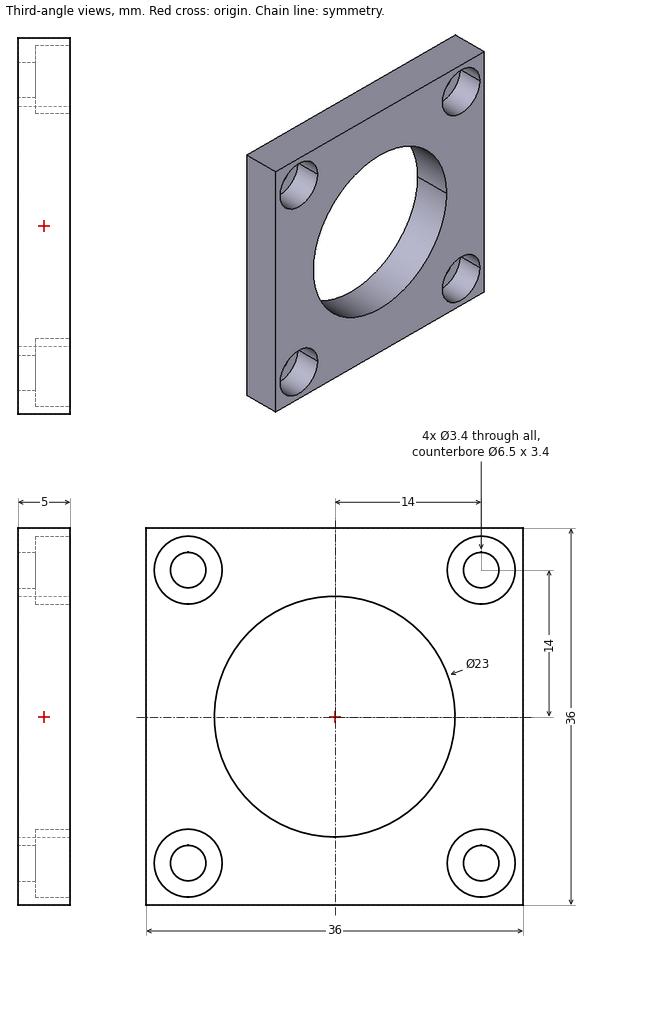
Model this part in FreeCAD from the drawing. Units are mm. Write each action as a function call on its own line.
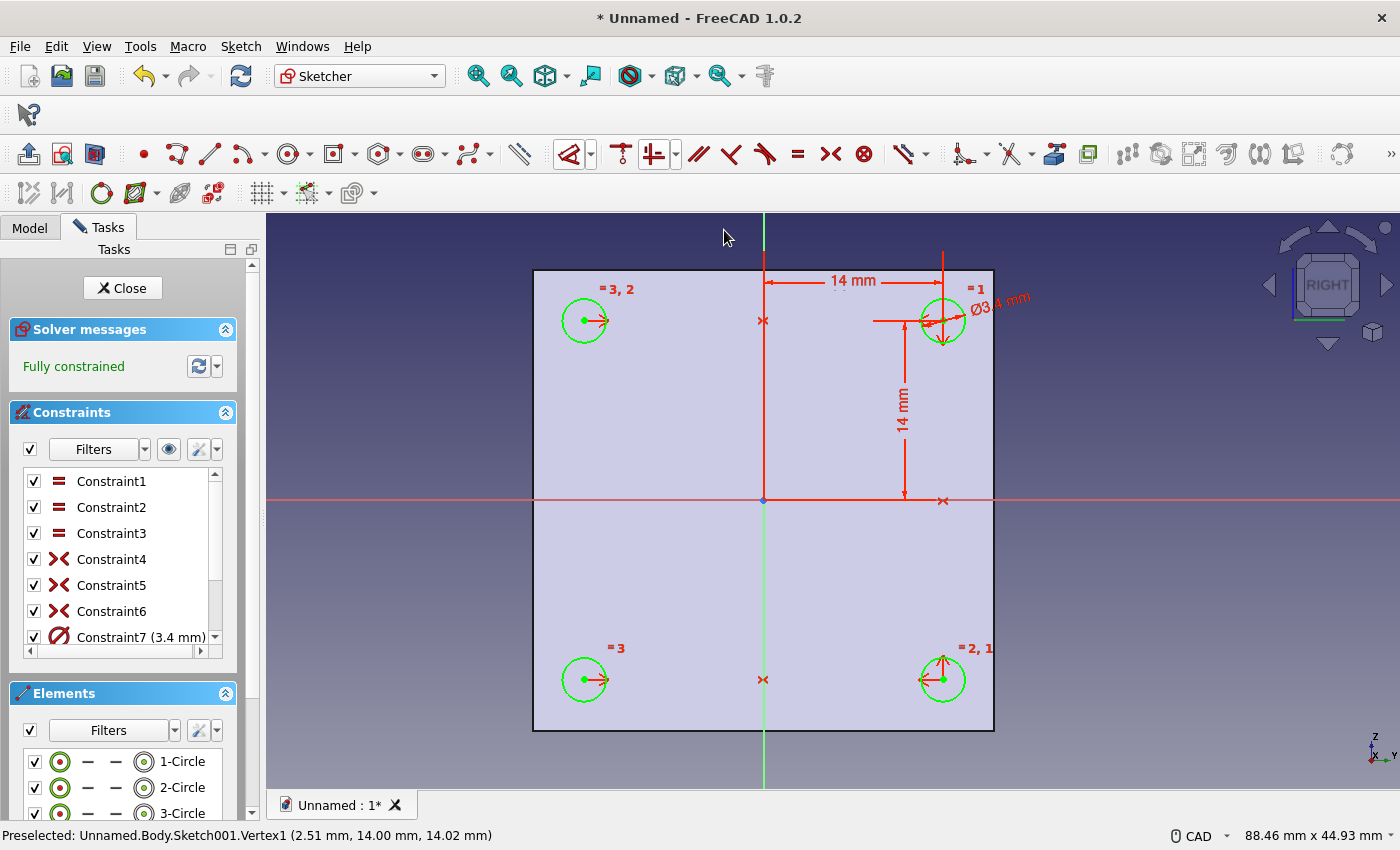
click(123, 288)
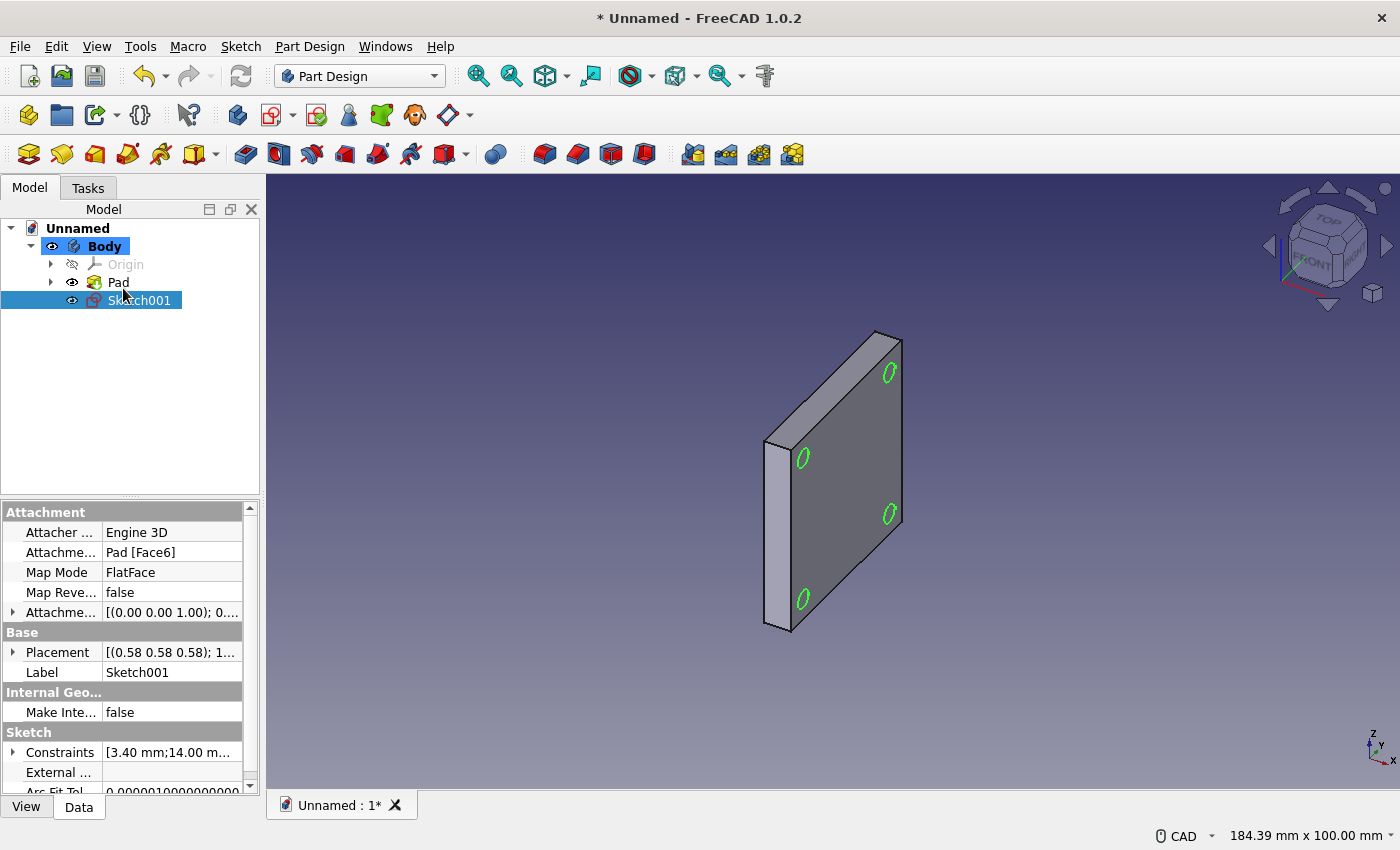
click(279, 154)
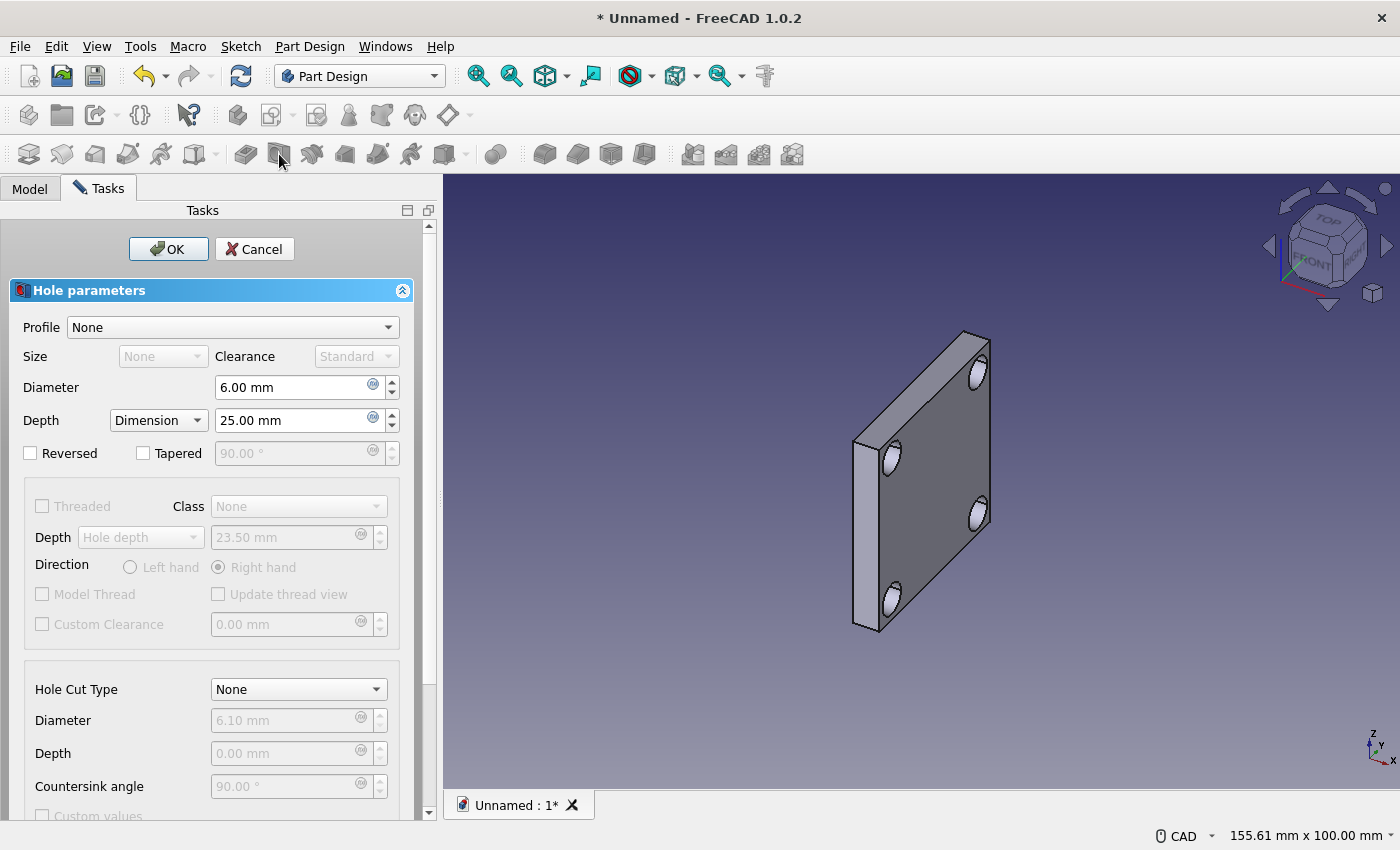
triple_click(300, 388)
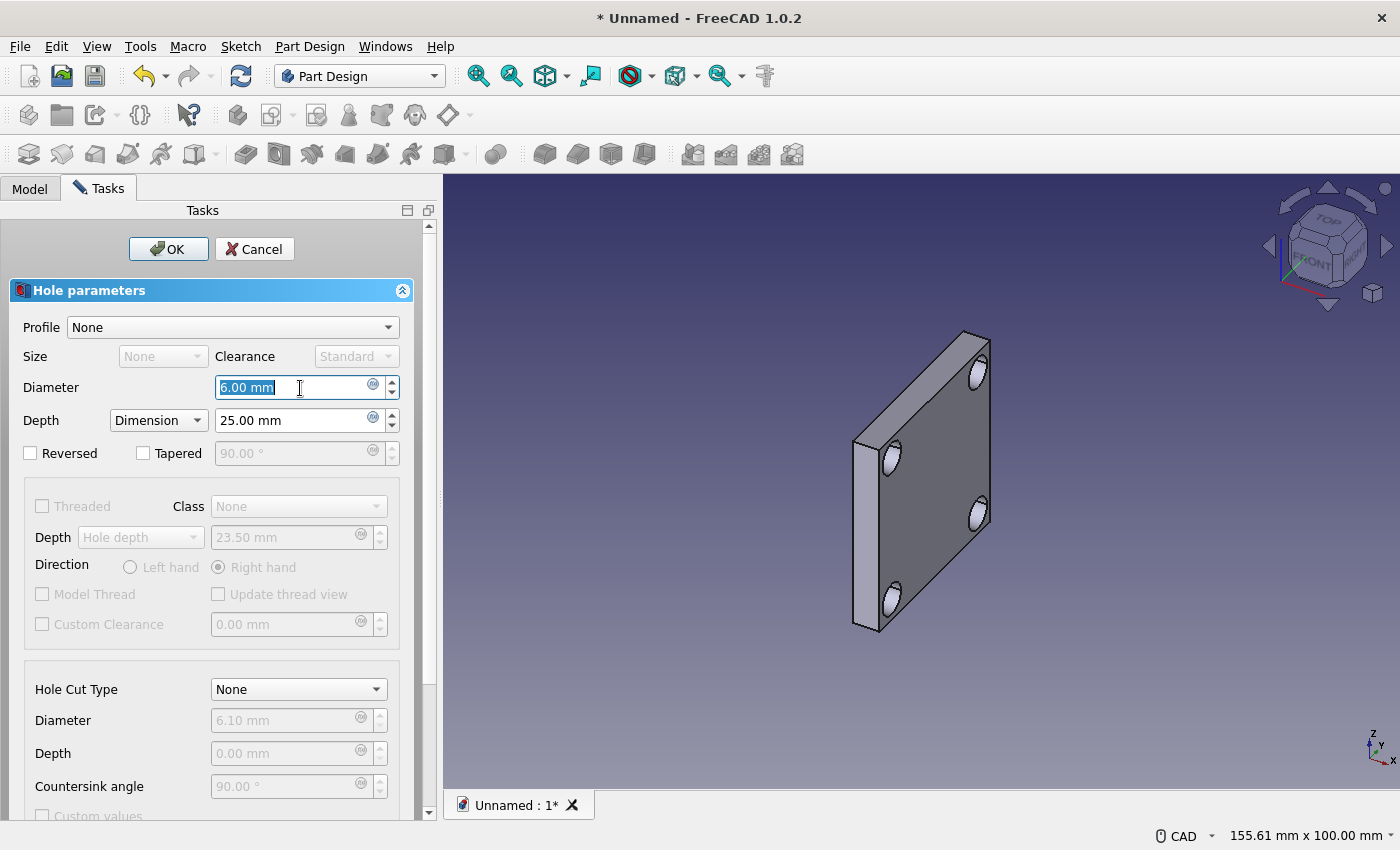
text(3.4)
key(Tab)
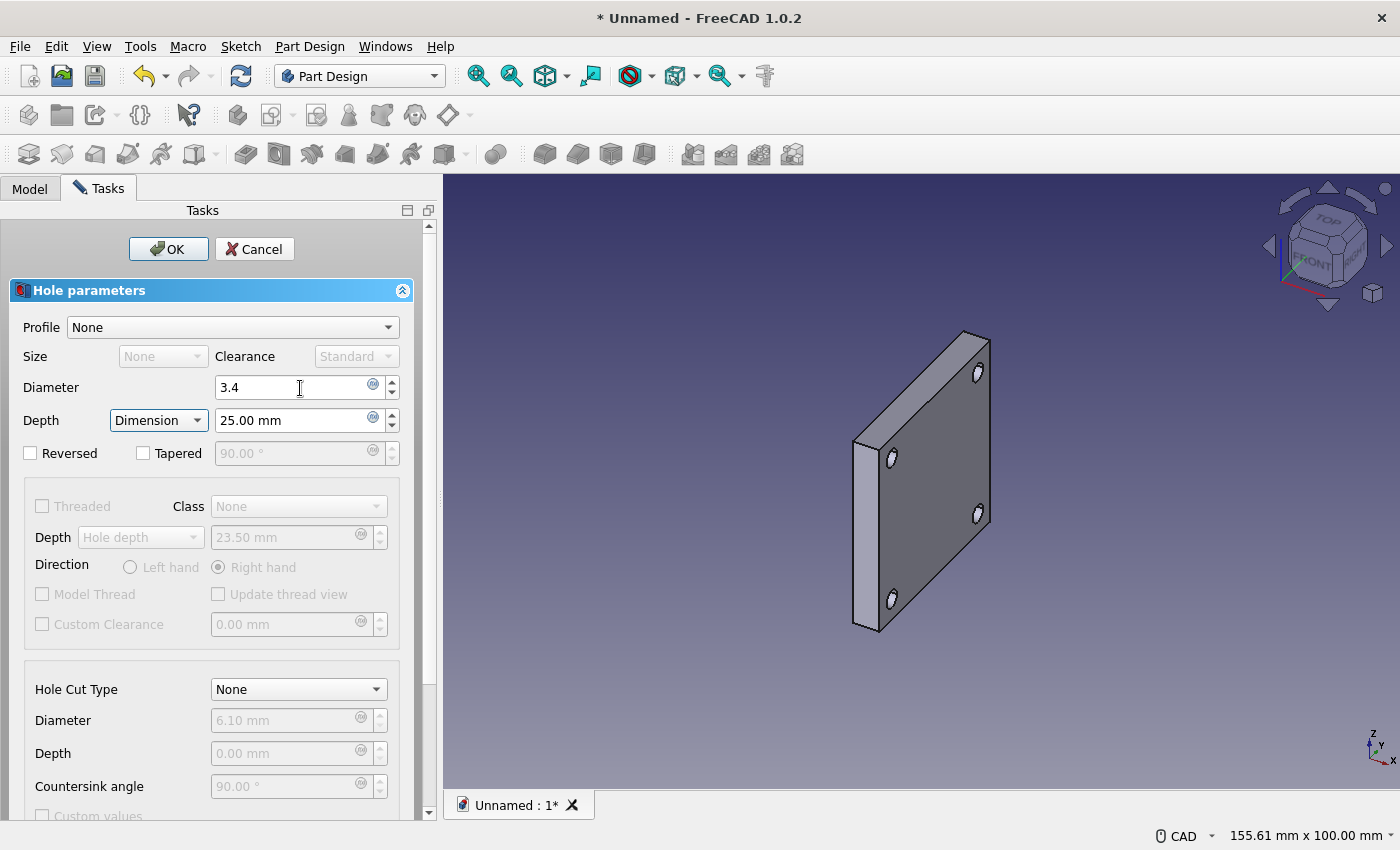
click(160, 420)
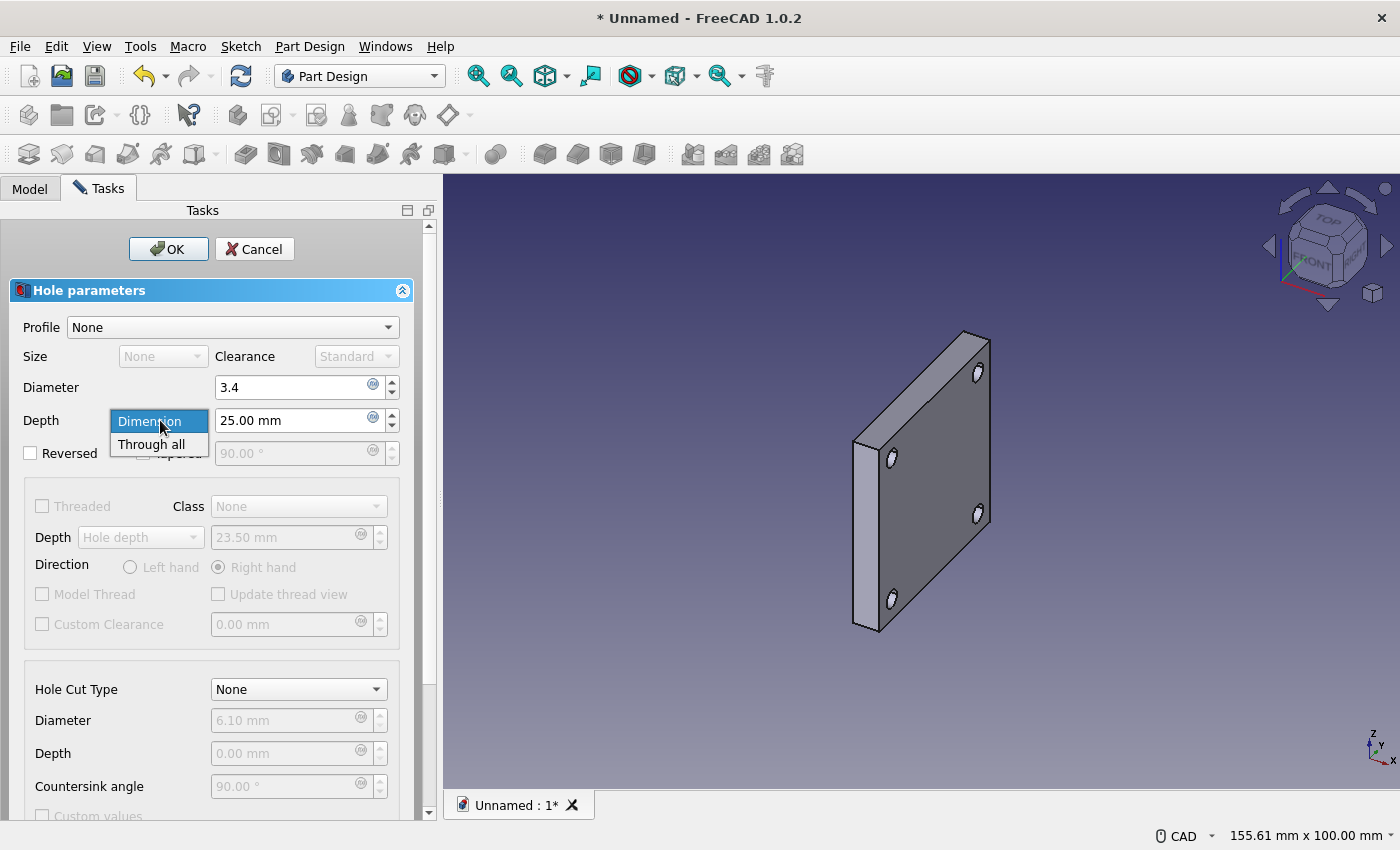
click(158, 444)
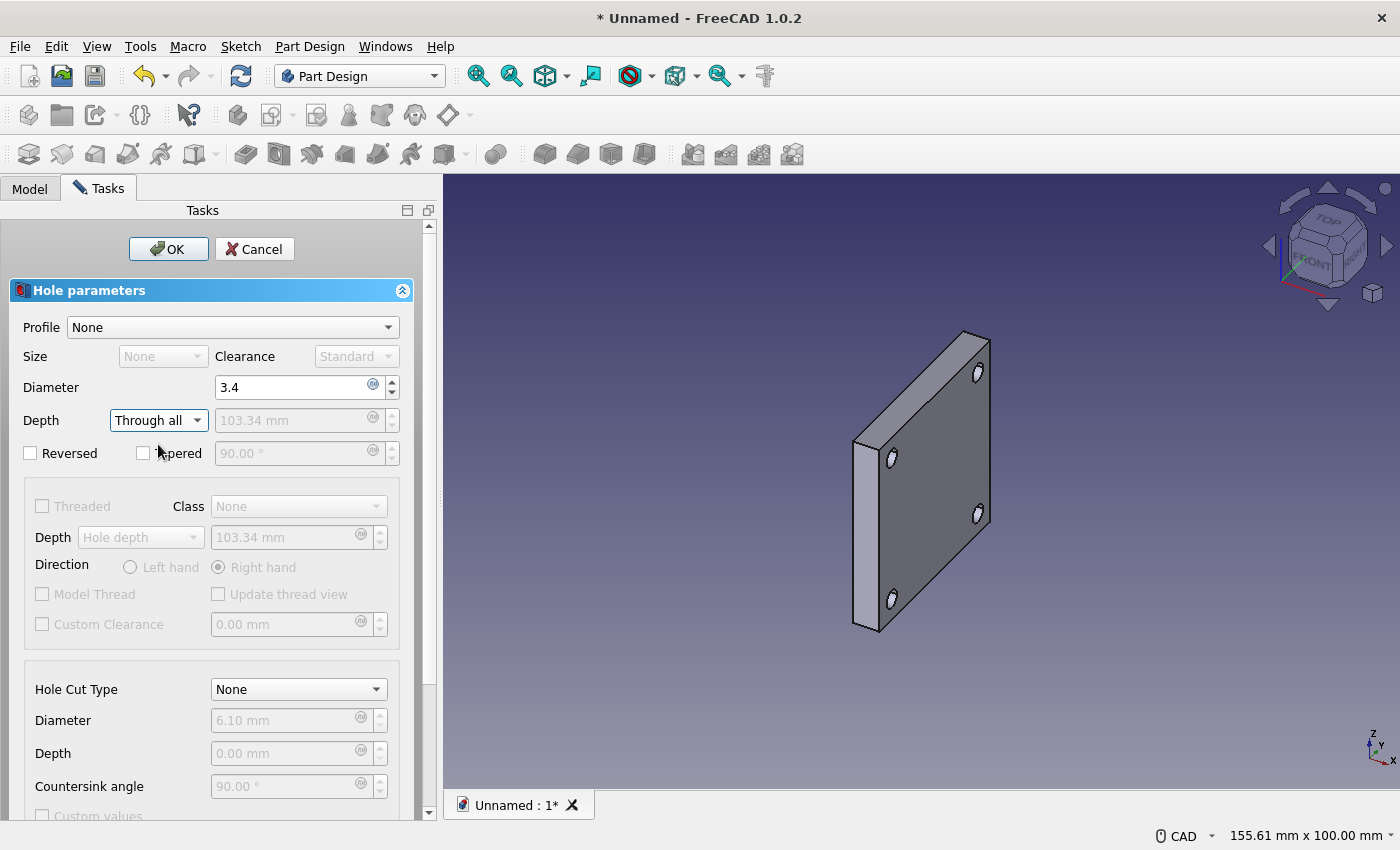
click(300, 690)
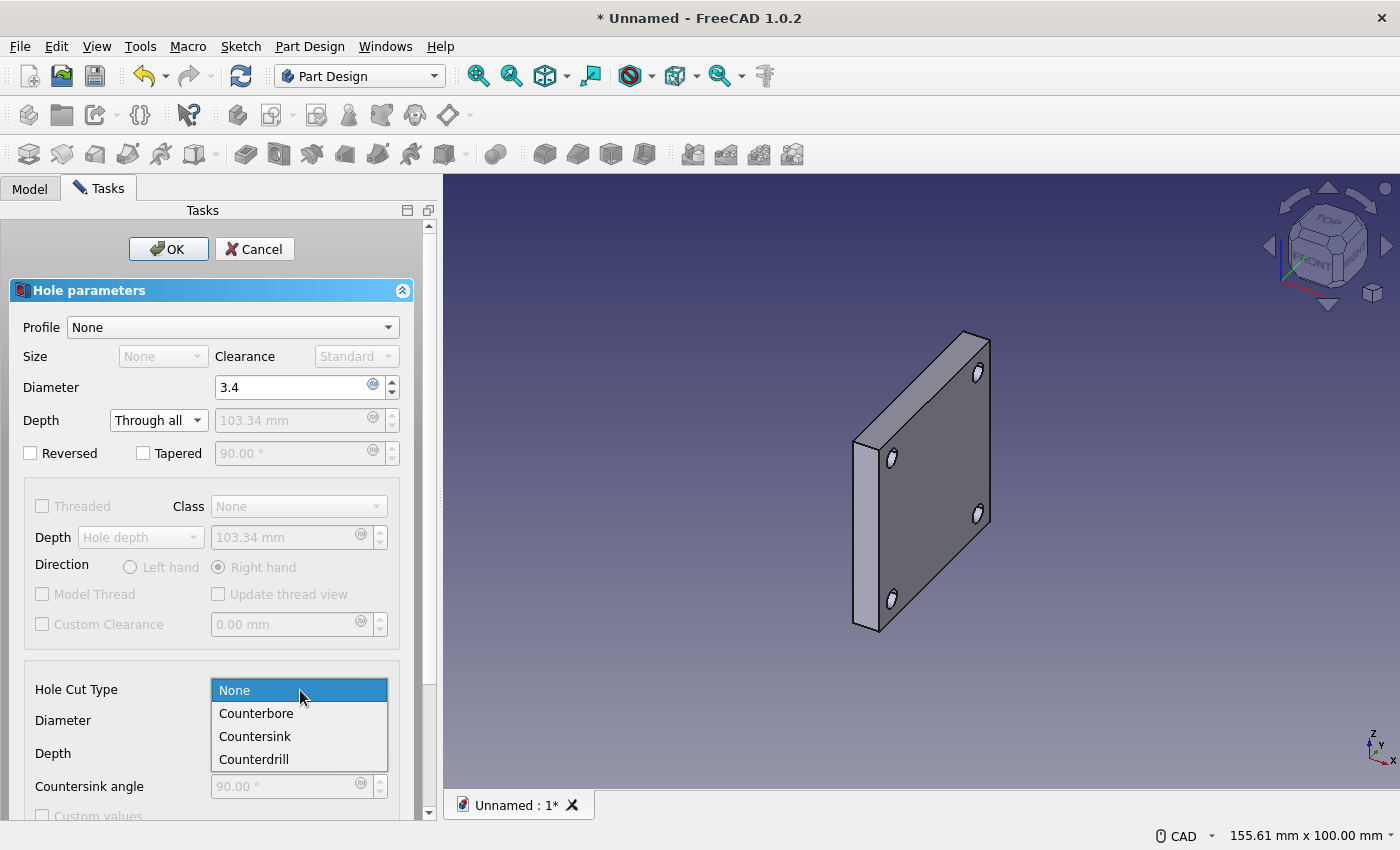
click(298, 714)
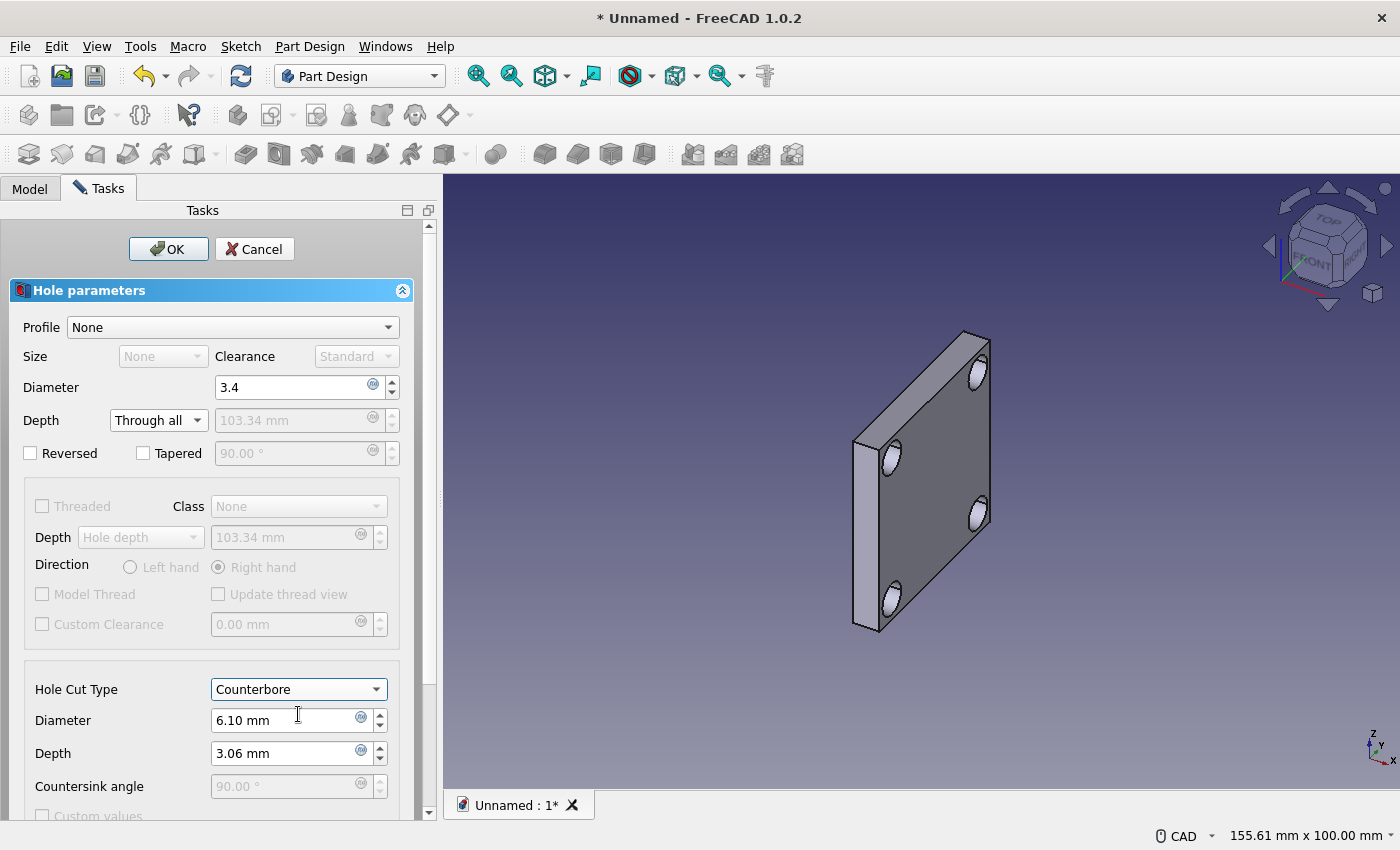
triple_click(292, 720)